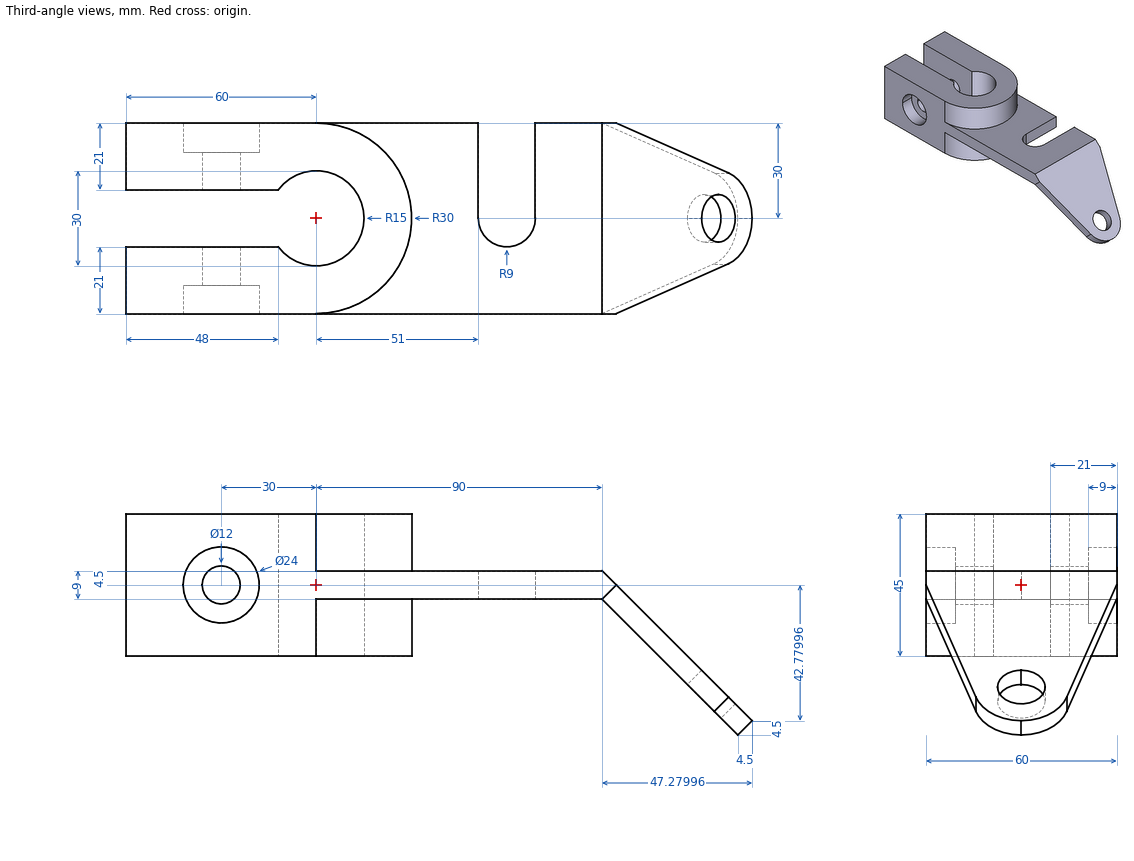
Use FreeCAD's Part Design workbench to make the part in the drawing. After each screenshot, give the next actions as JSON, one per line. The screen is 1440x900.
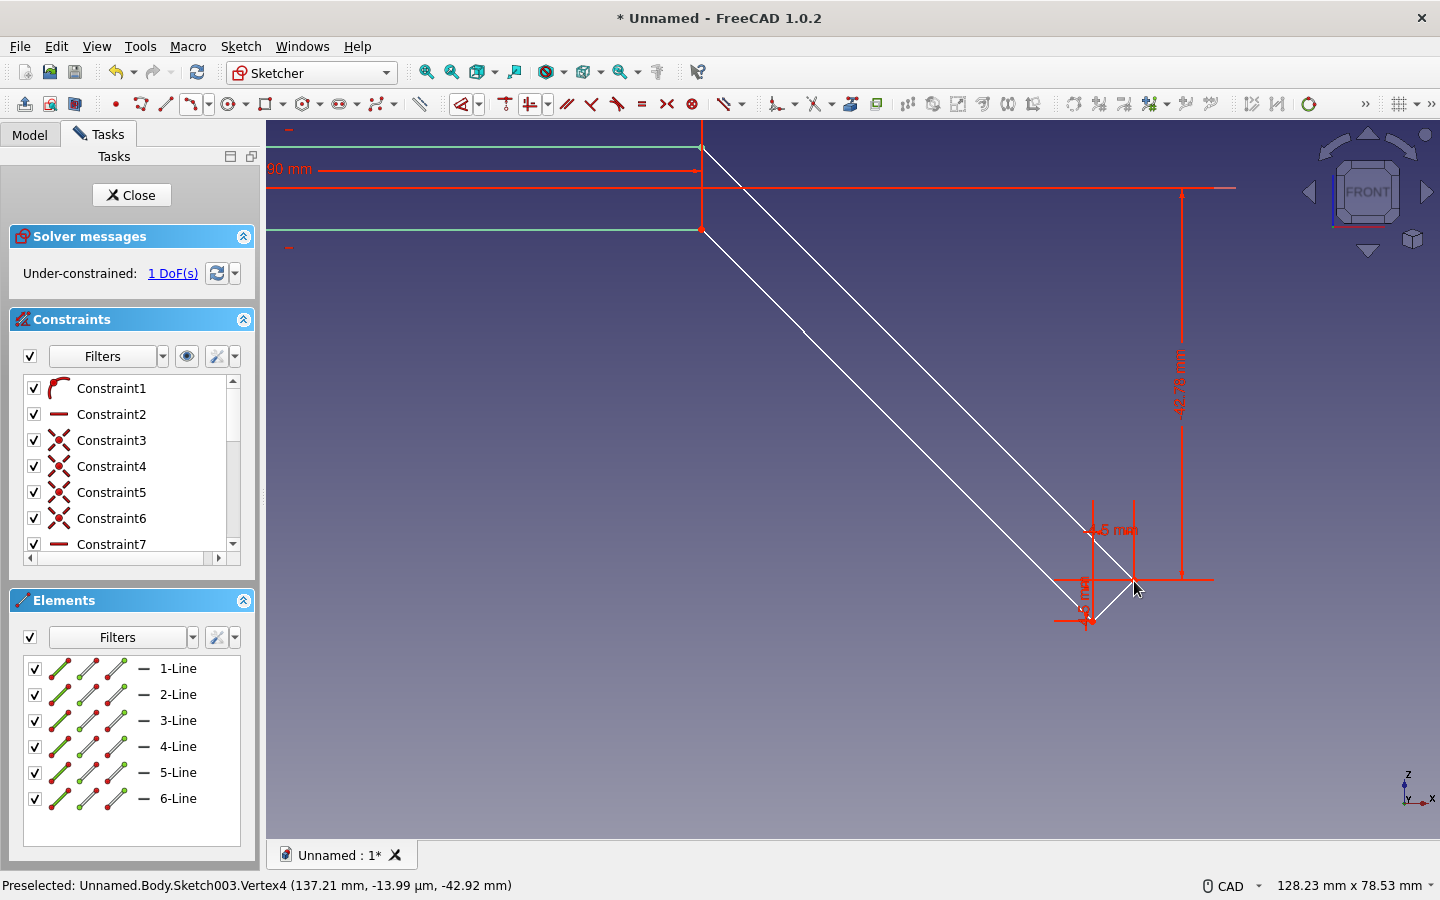
{"action": "left_click", "coordinate": [831, 277]}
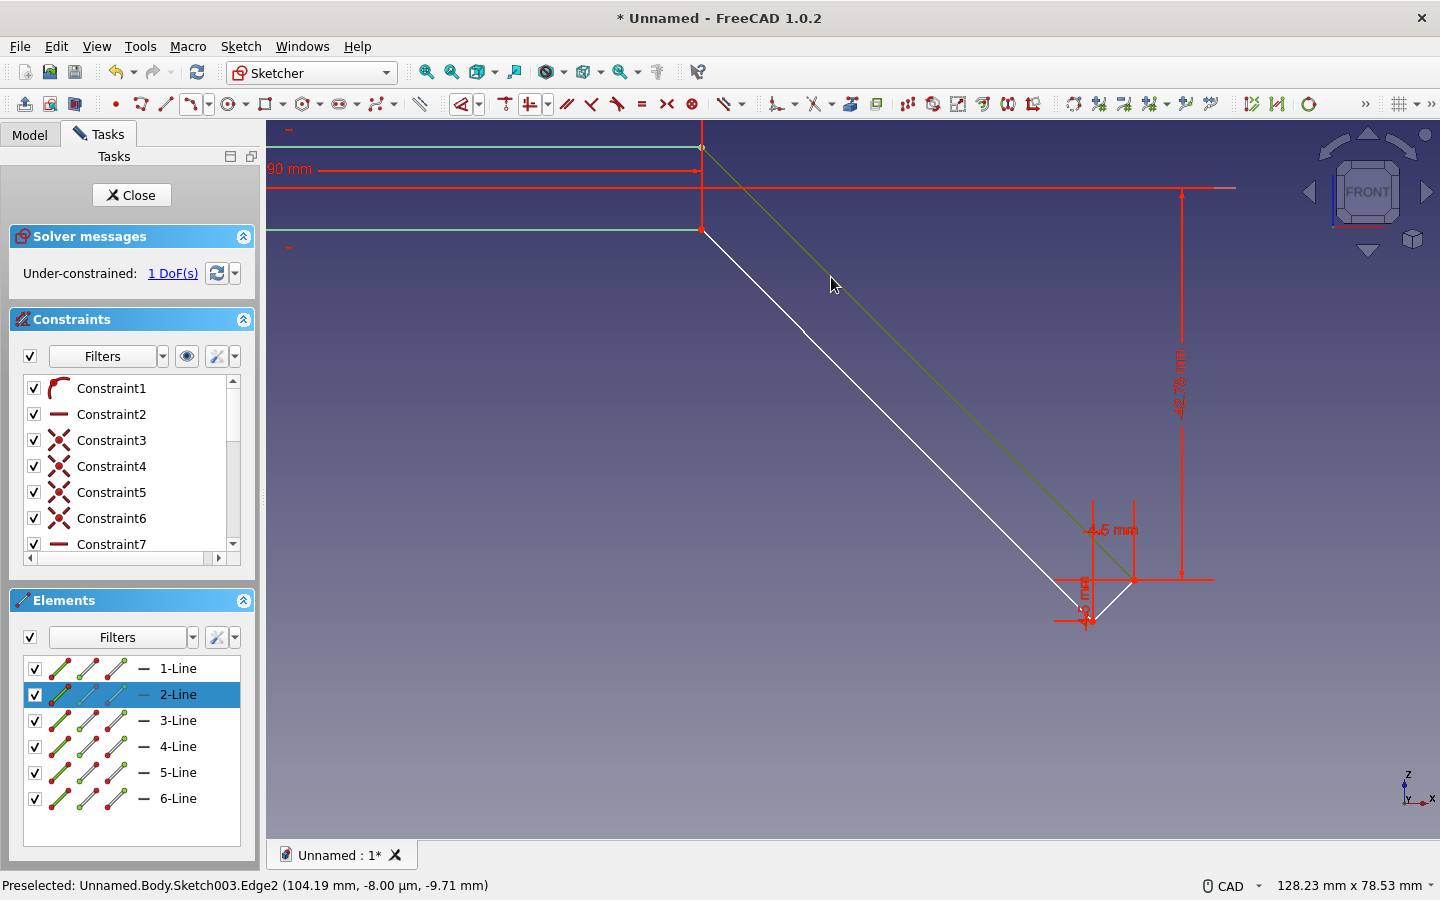
{"action": "key", "text": "l"}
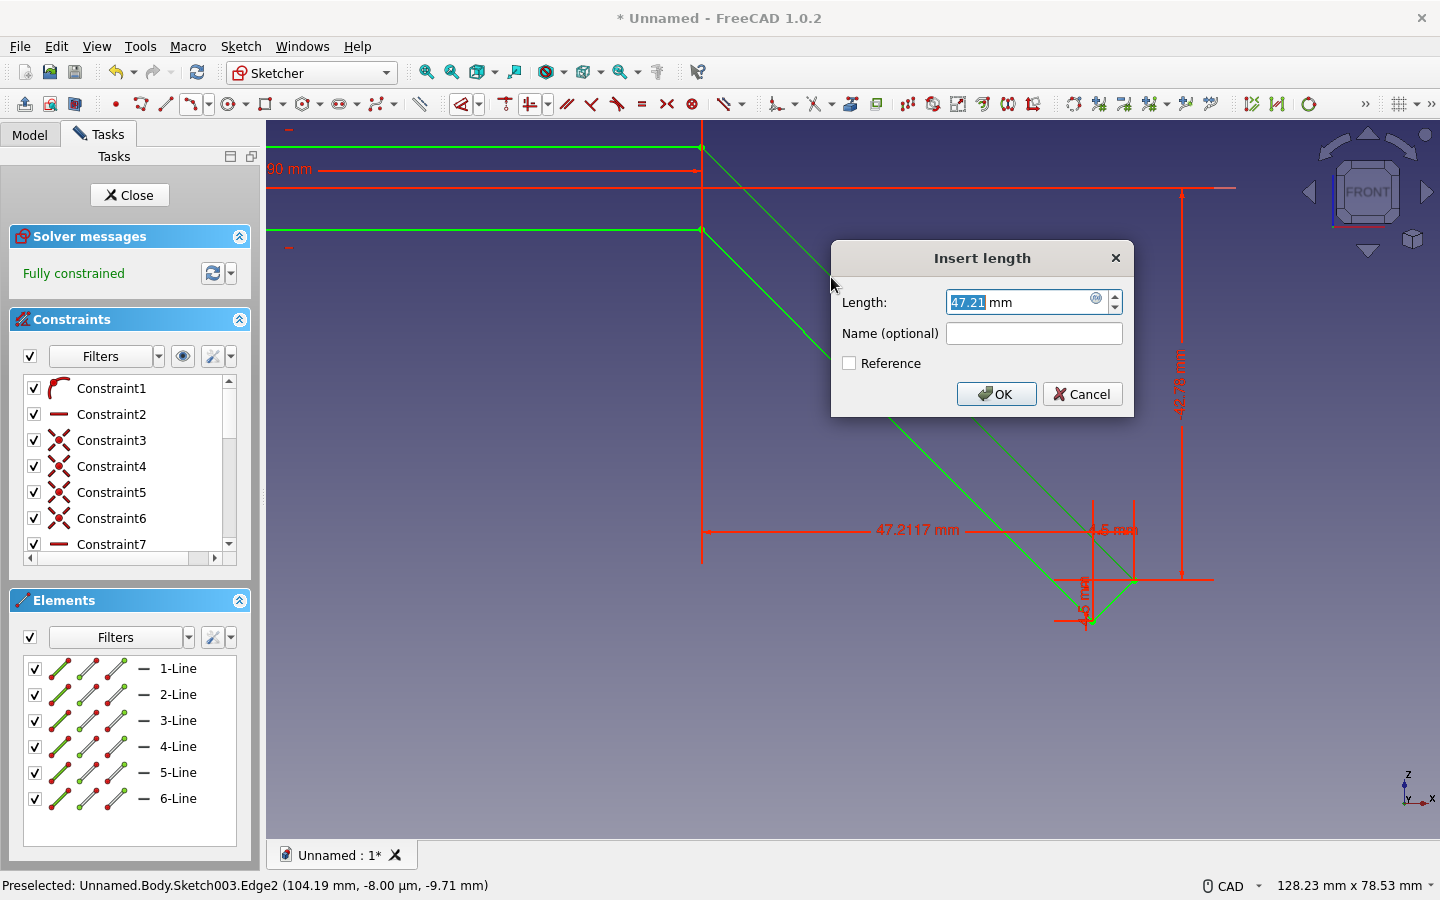
{"action": "type", "text": "47.27996"}
{"action": "key", "text": "Return"}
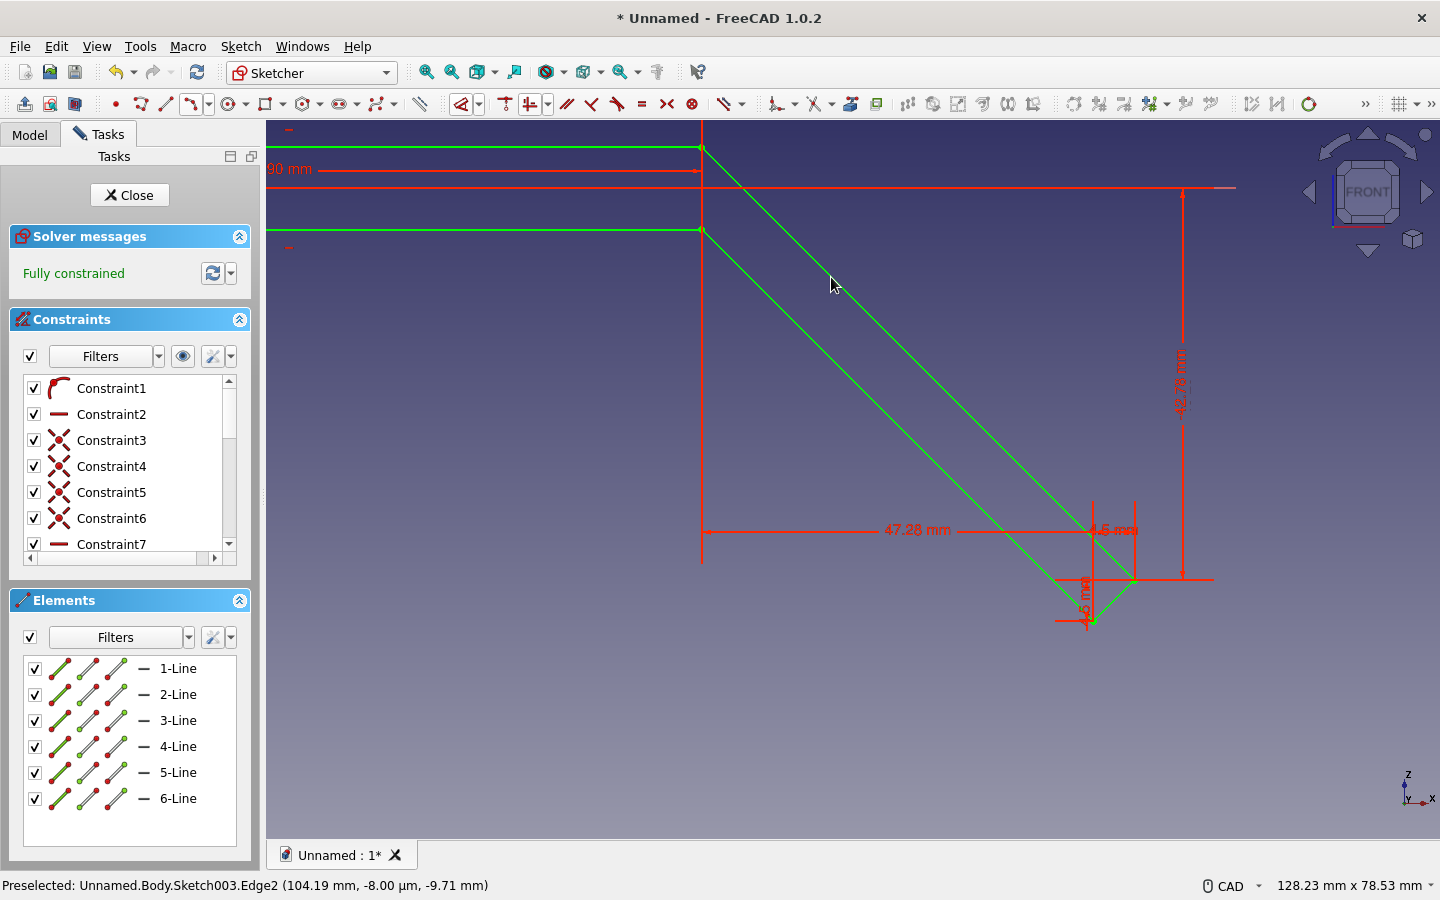
{"action": "left_click", "coordinate": [130, 195]}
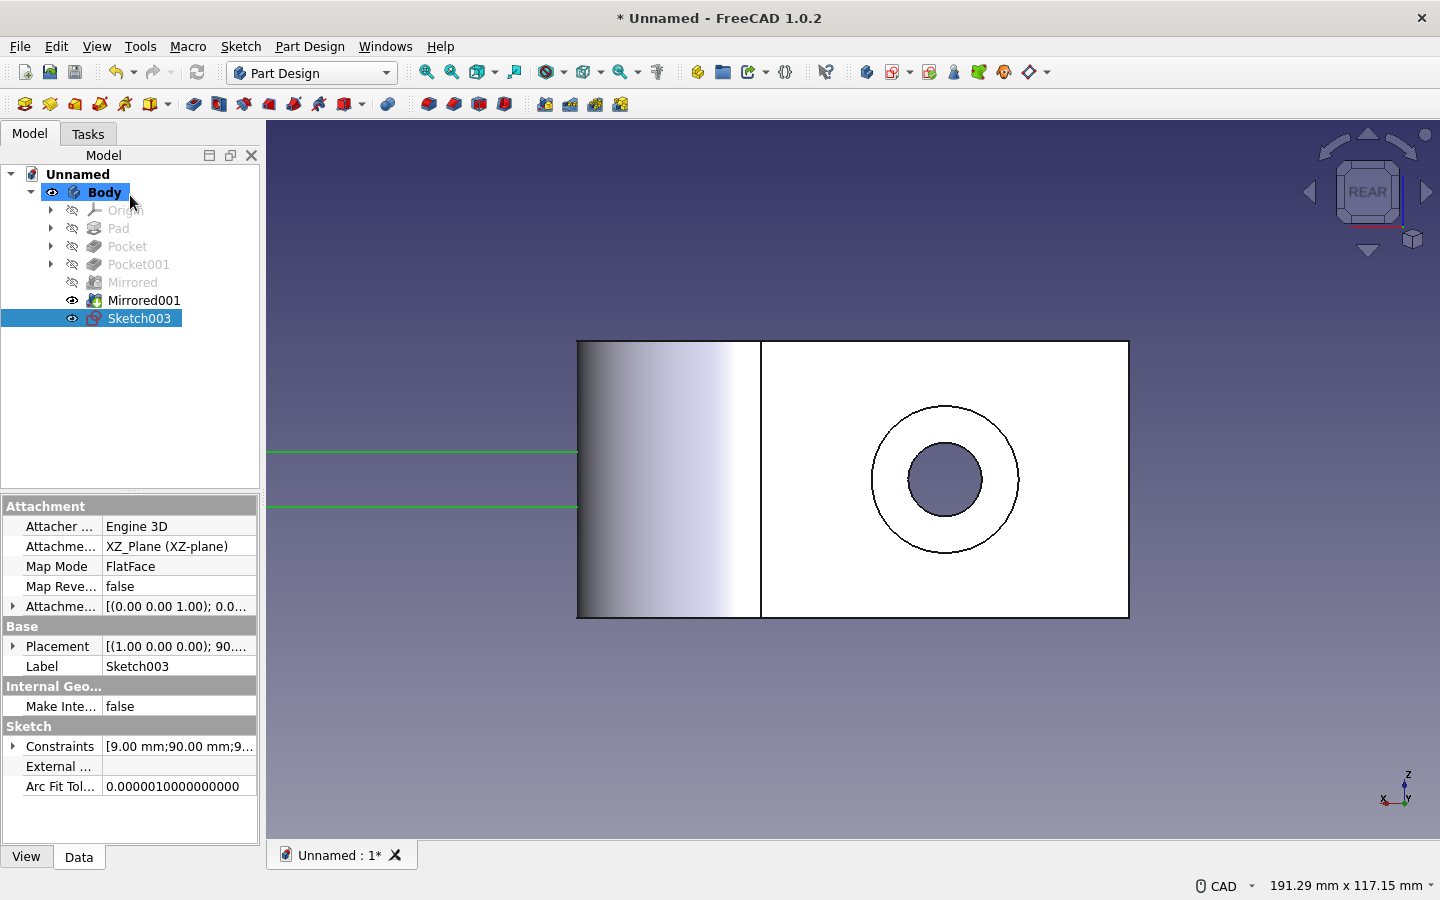
{"action": "left_click", "coordinate": [25, 104]}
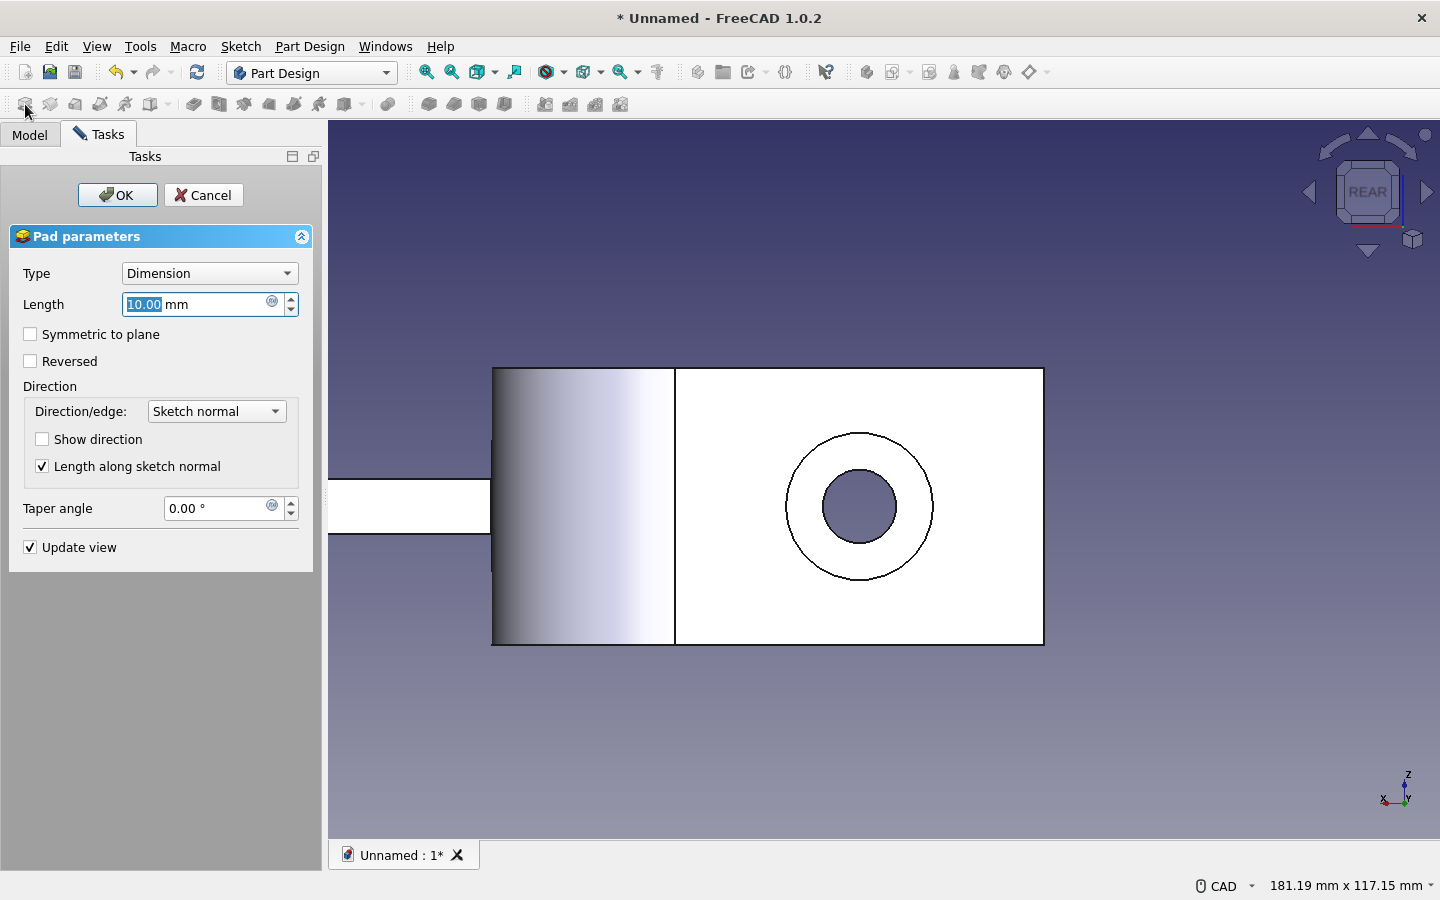
{"action": "type", "text": "60"}
{"action": "key", "text": "Tab"}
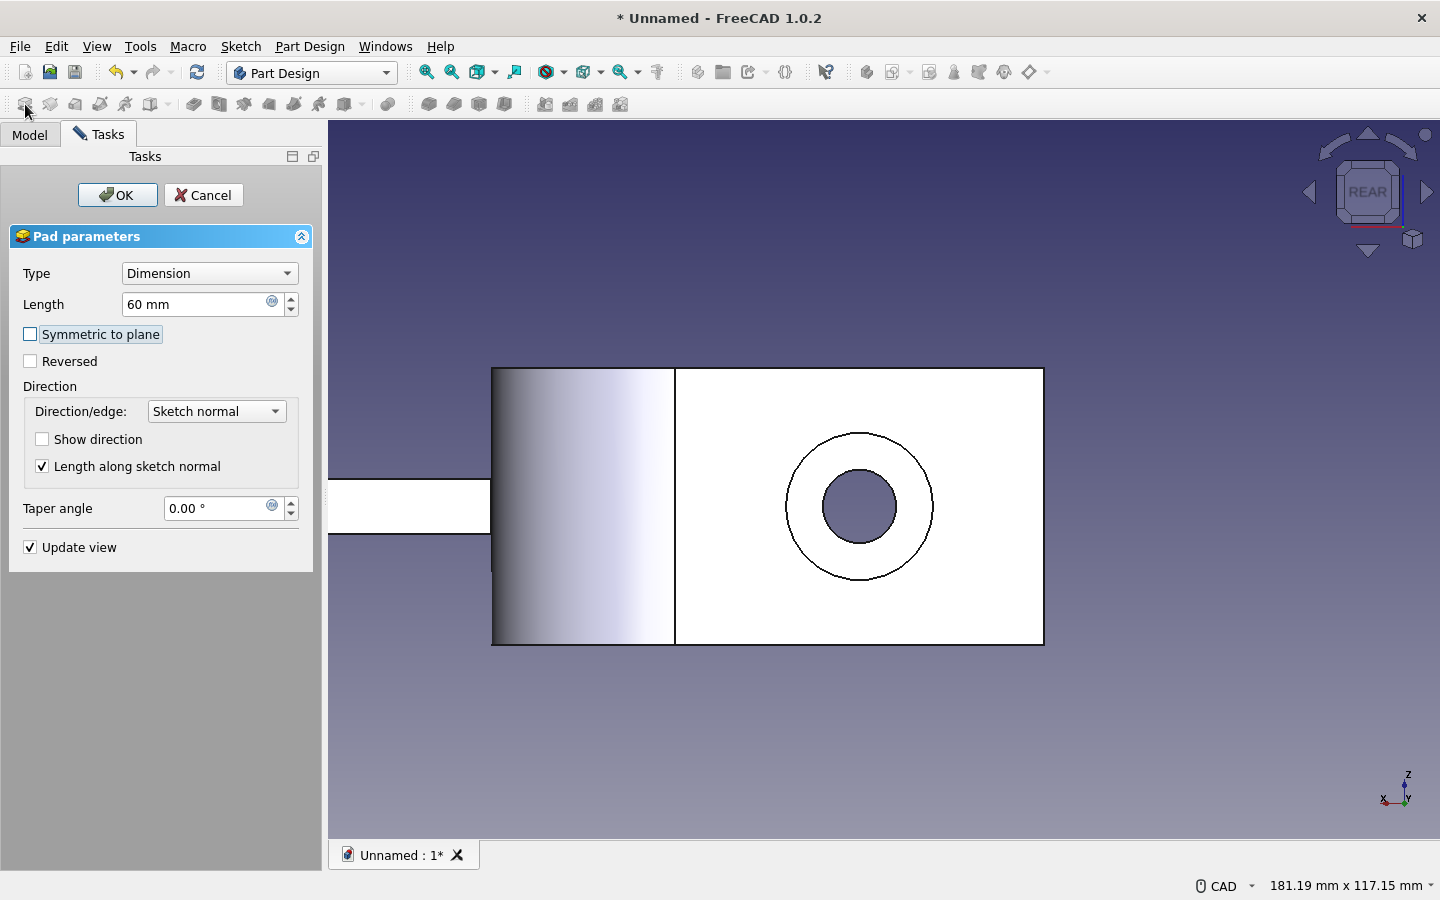
{"action": "left_click", "coordinate": [31, 334]}